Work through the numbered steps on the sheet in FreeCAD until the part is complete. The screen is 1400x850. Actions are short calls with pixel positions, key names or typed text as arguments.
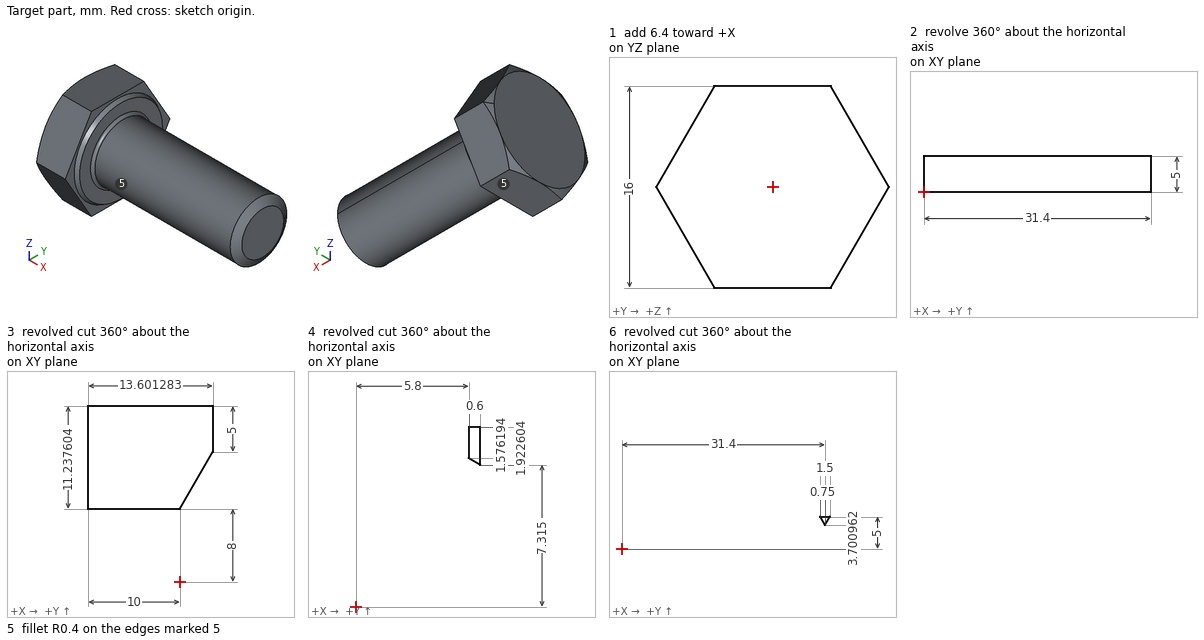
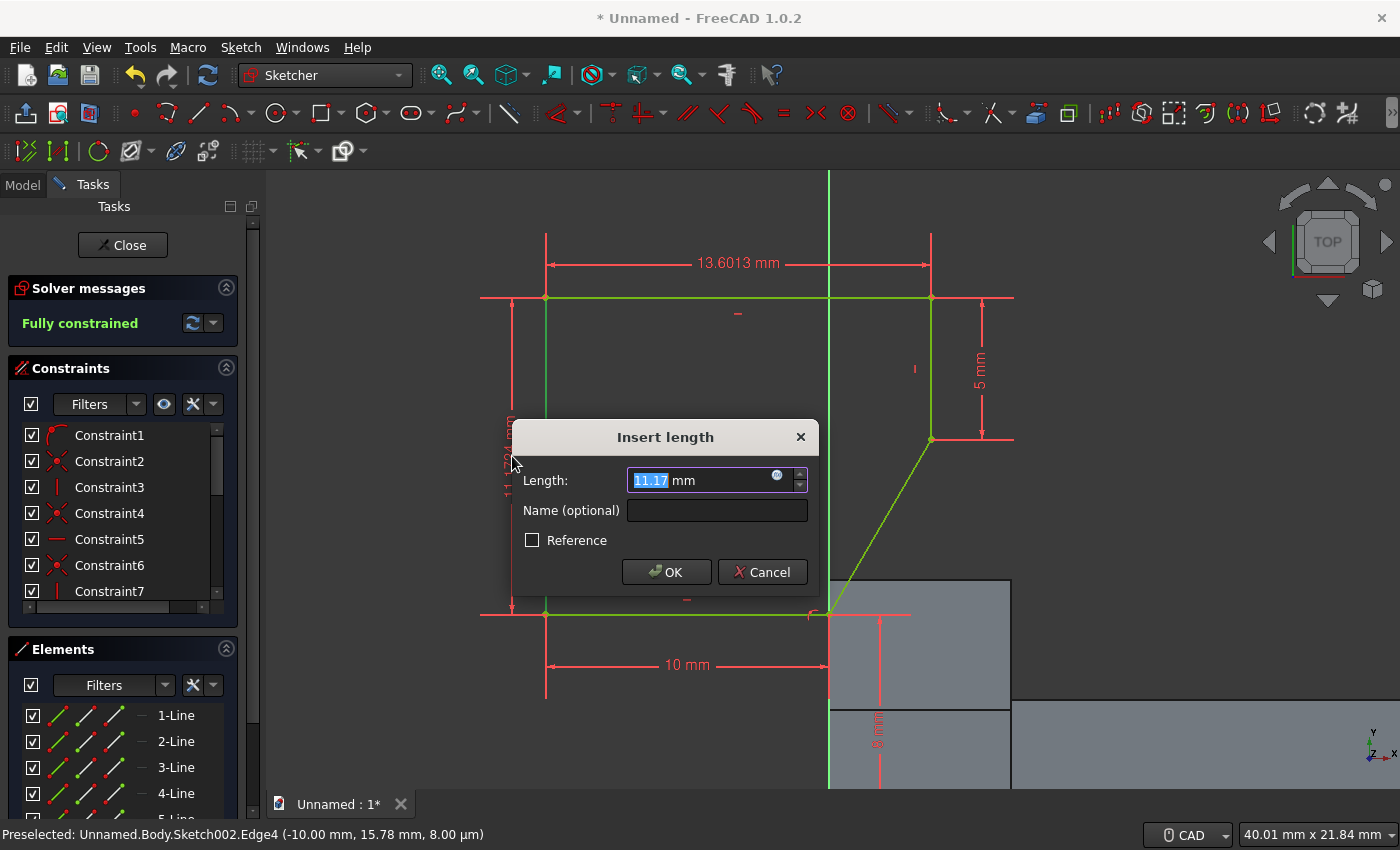
text(11.237604)
key(Return)
key(Escape)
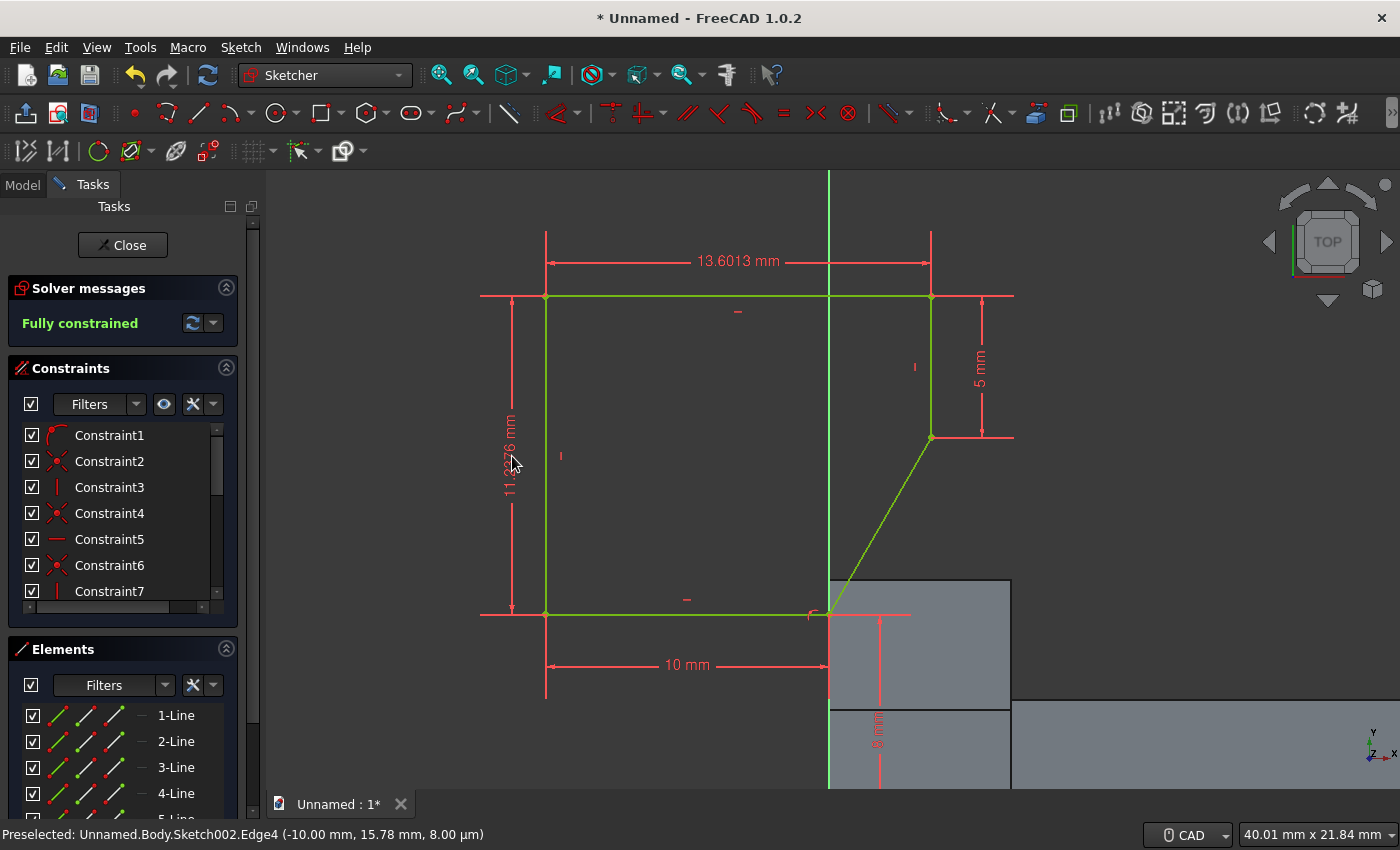
click(123, 245)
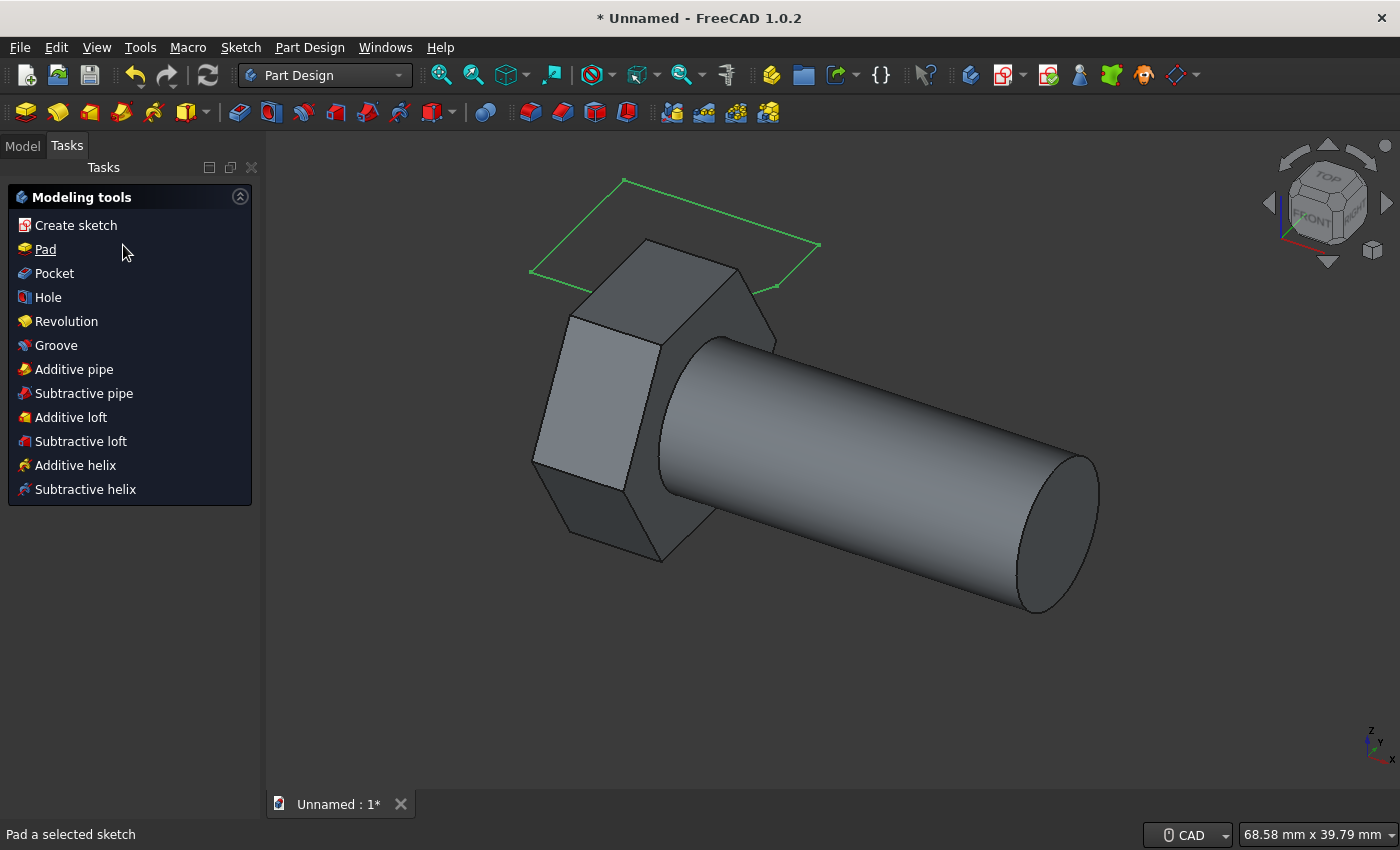
click(304, 112)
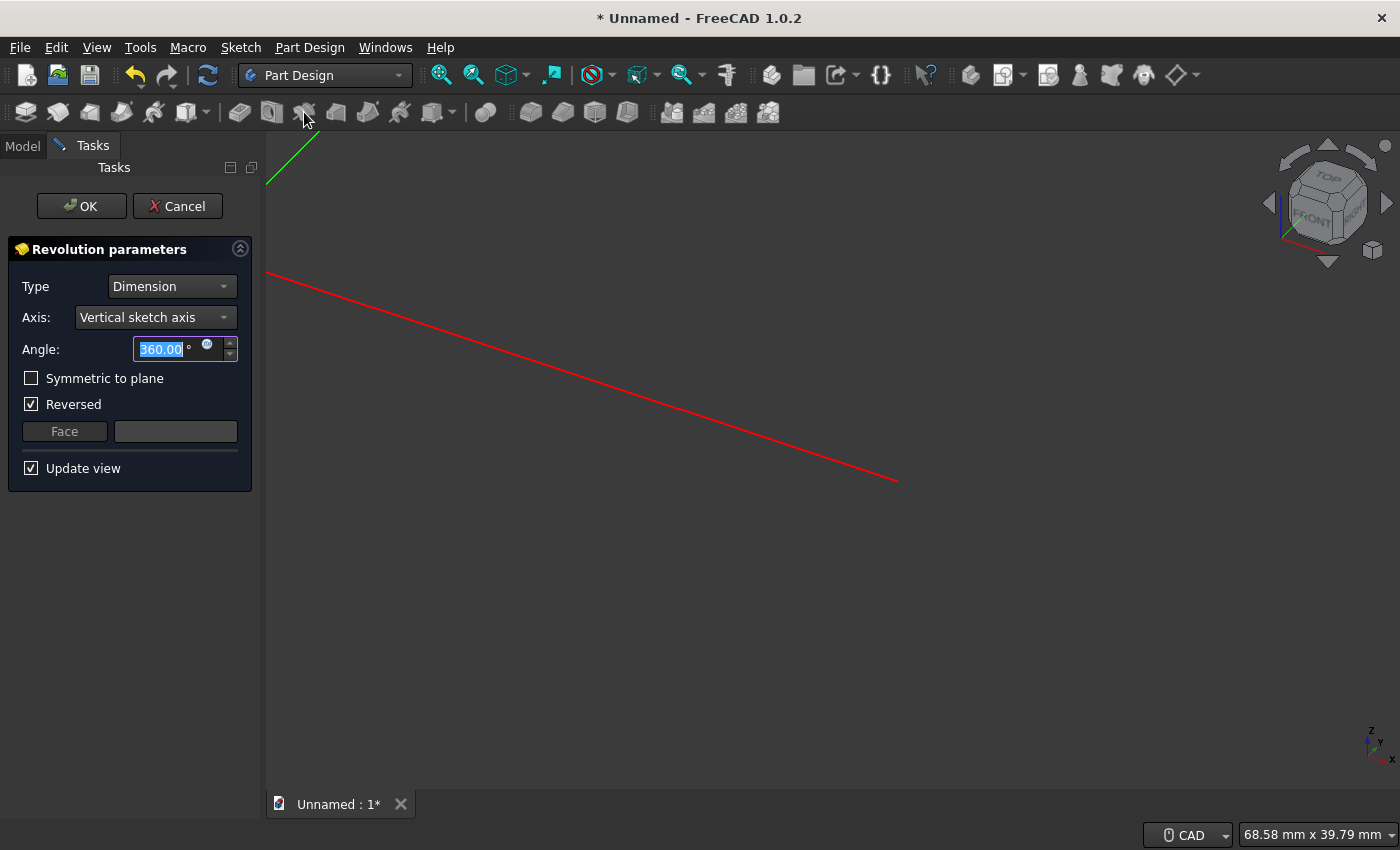
click(156, 318)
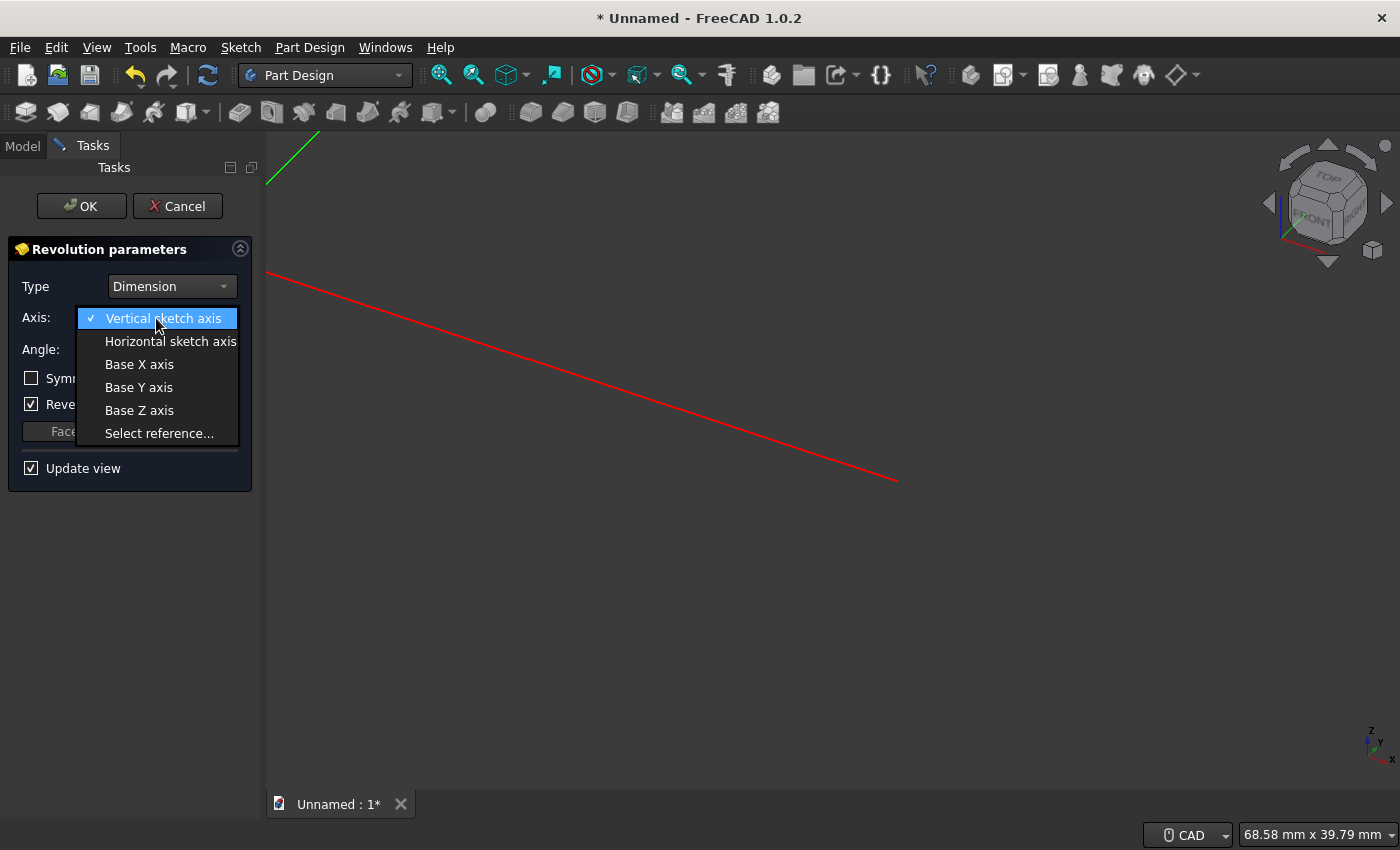
click(156, 342)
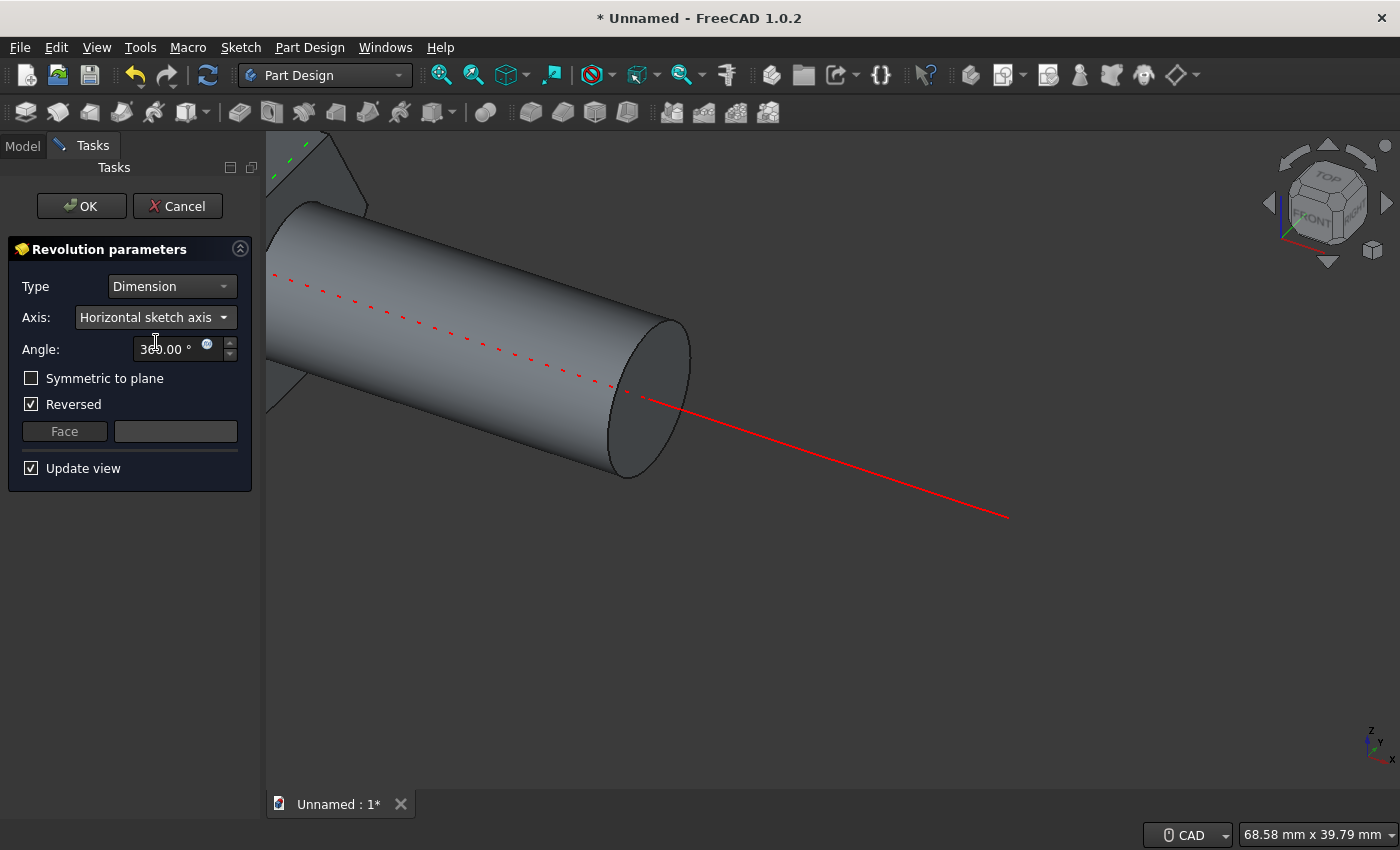
click(82, 206)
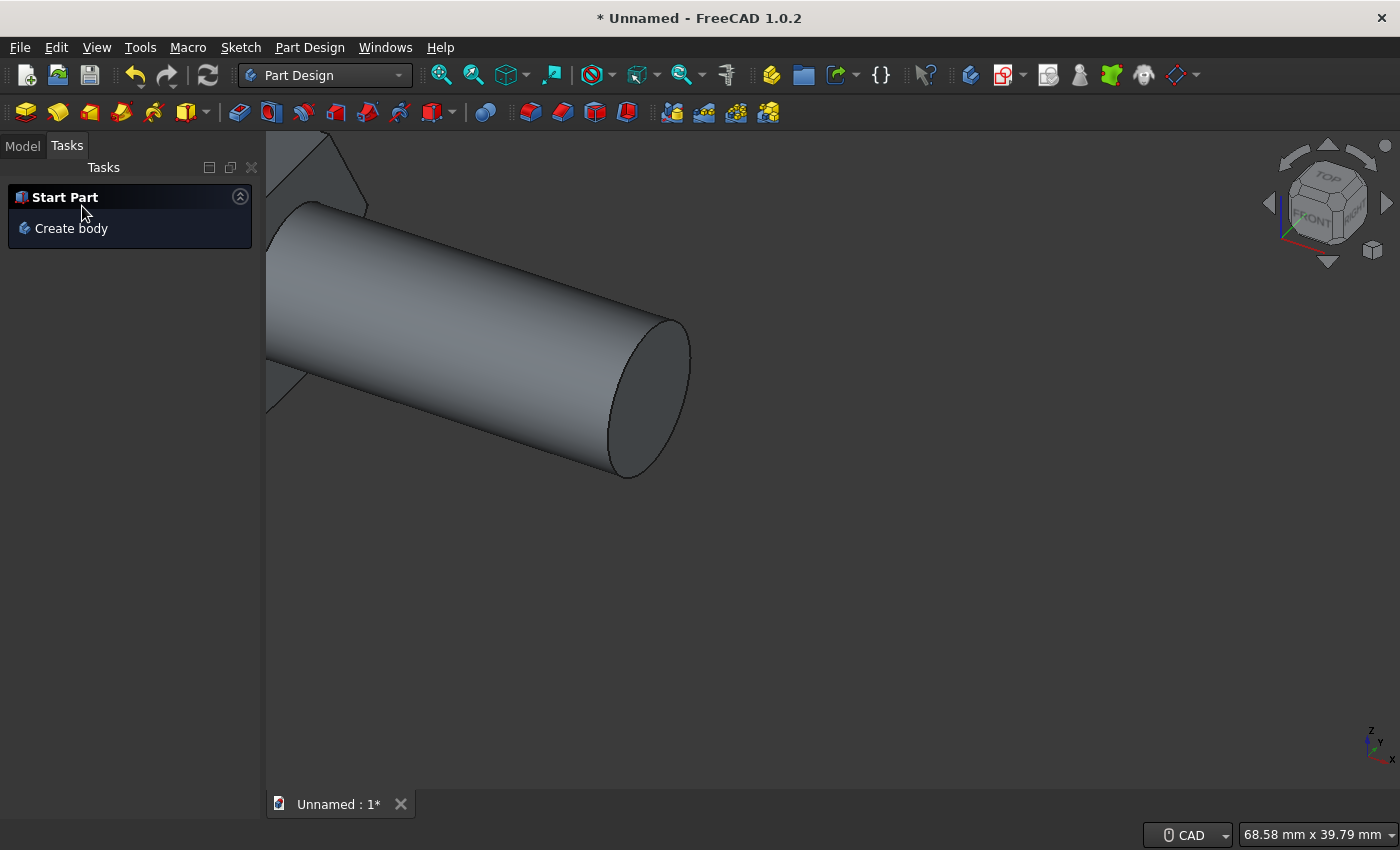
click(442, 76)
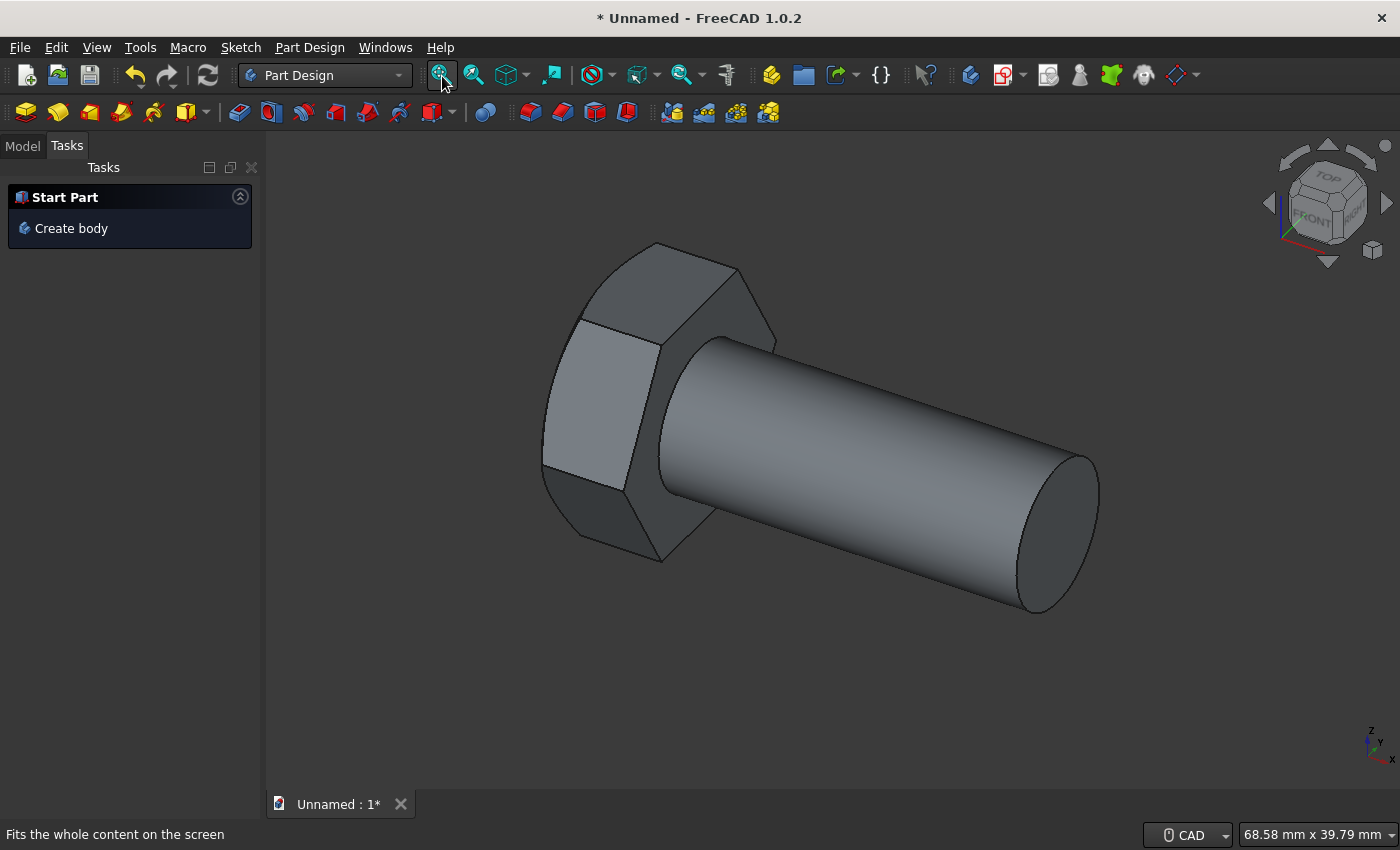
click(1004, 76)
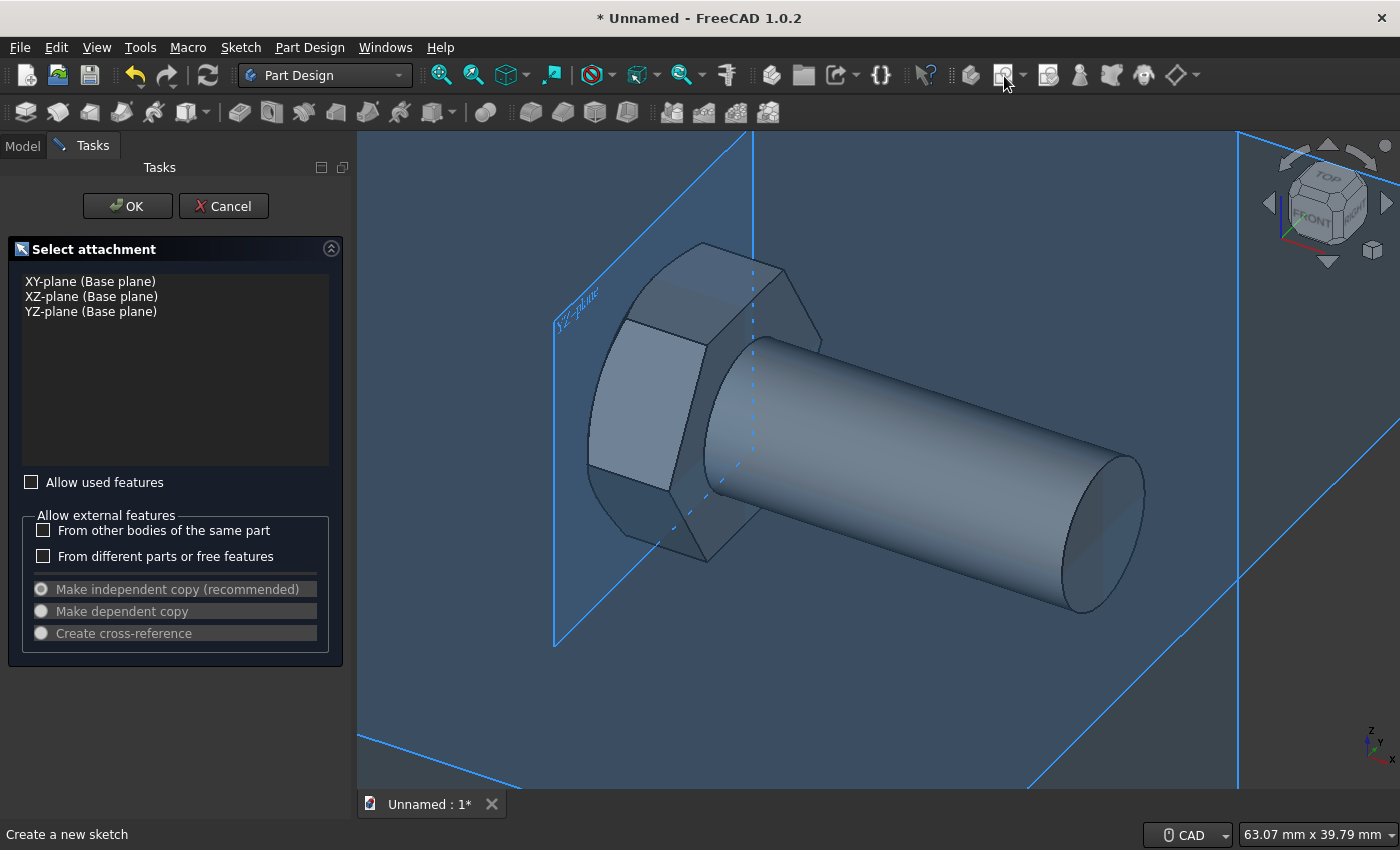
click(82, 282)